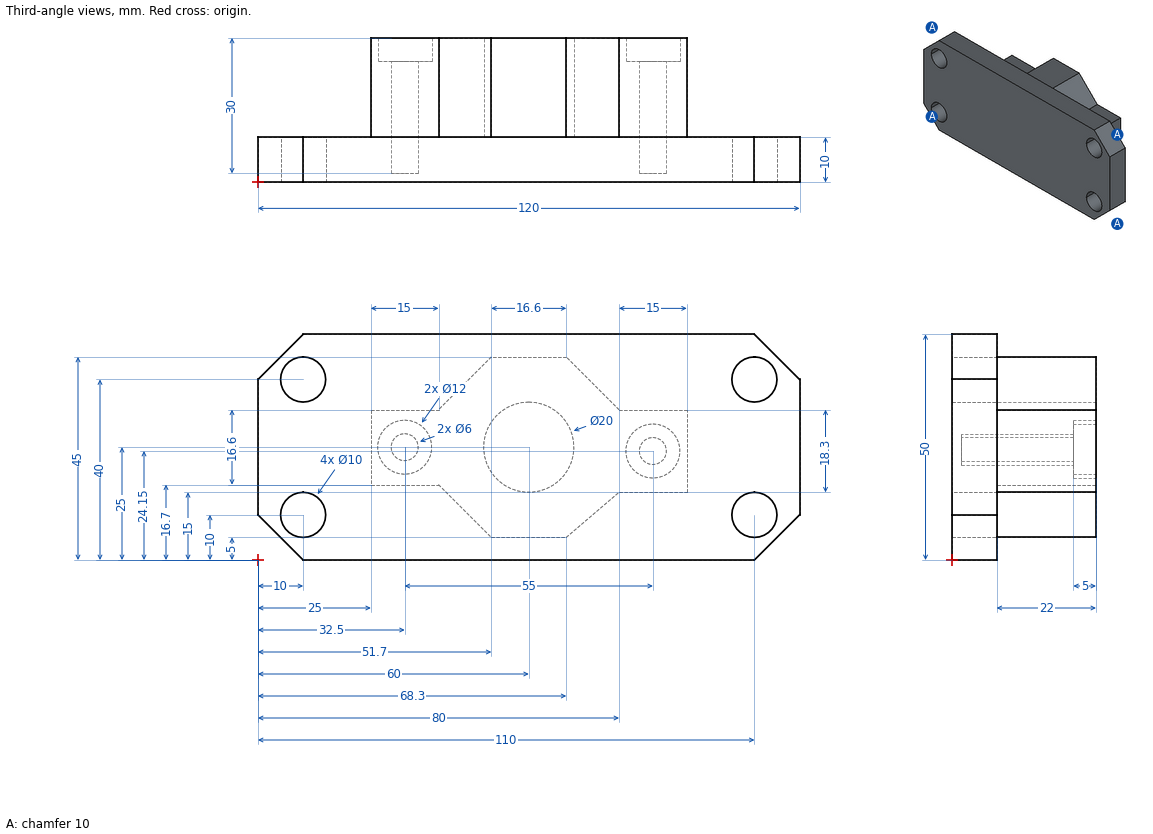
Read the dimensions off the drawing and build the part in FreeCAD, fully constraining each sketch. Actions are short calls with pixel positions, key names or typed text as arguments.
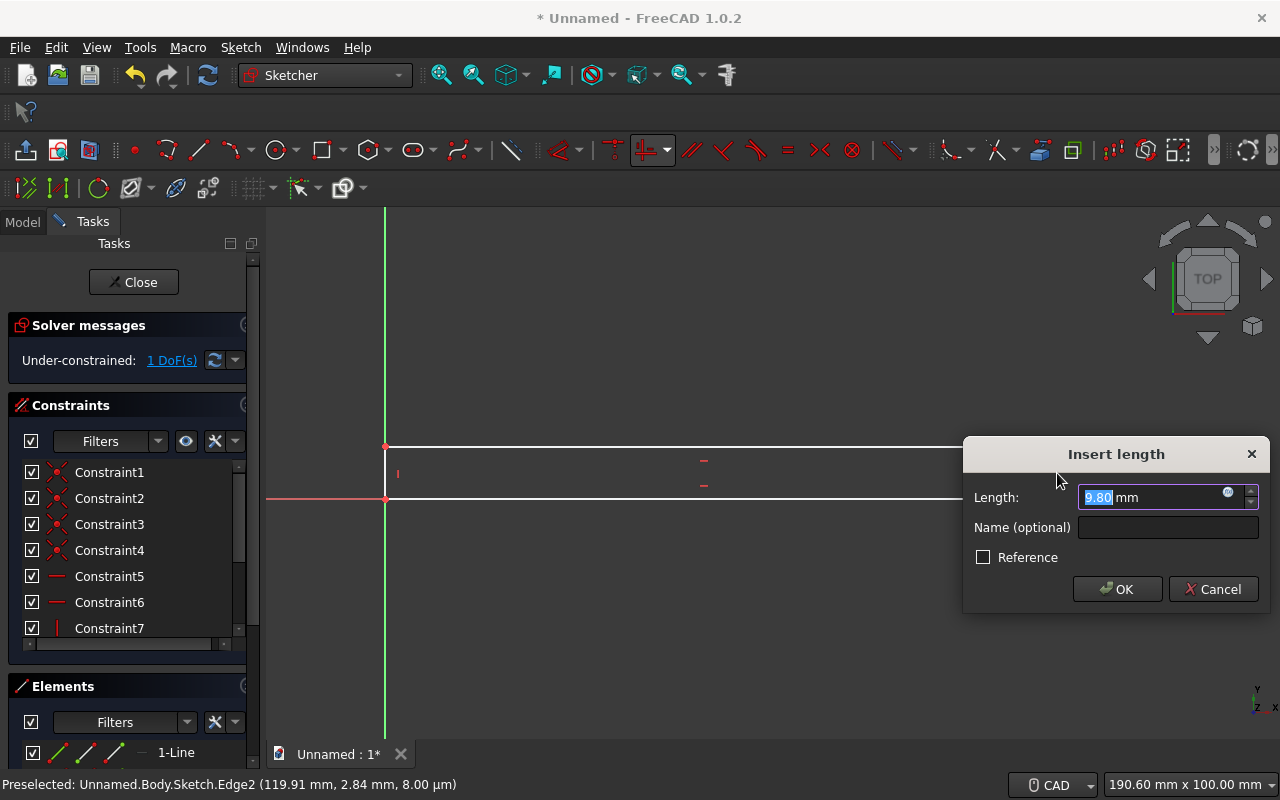
text(10)
key(Return)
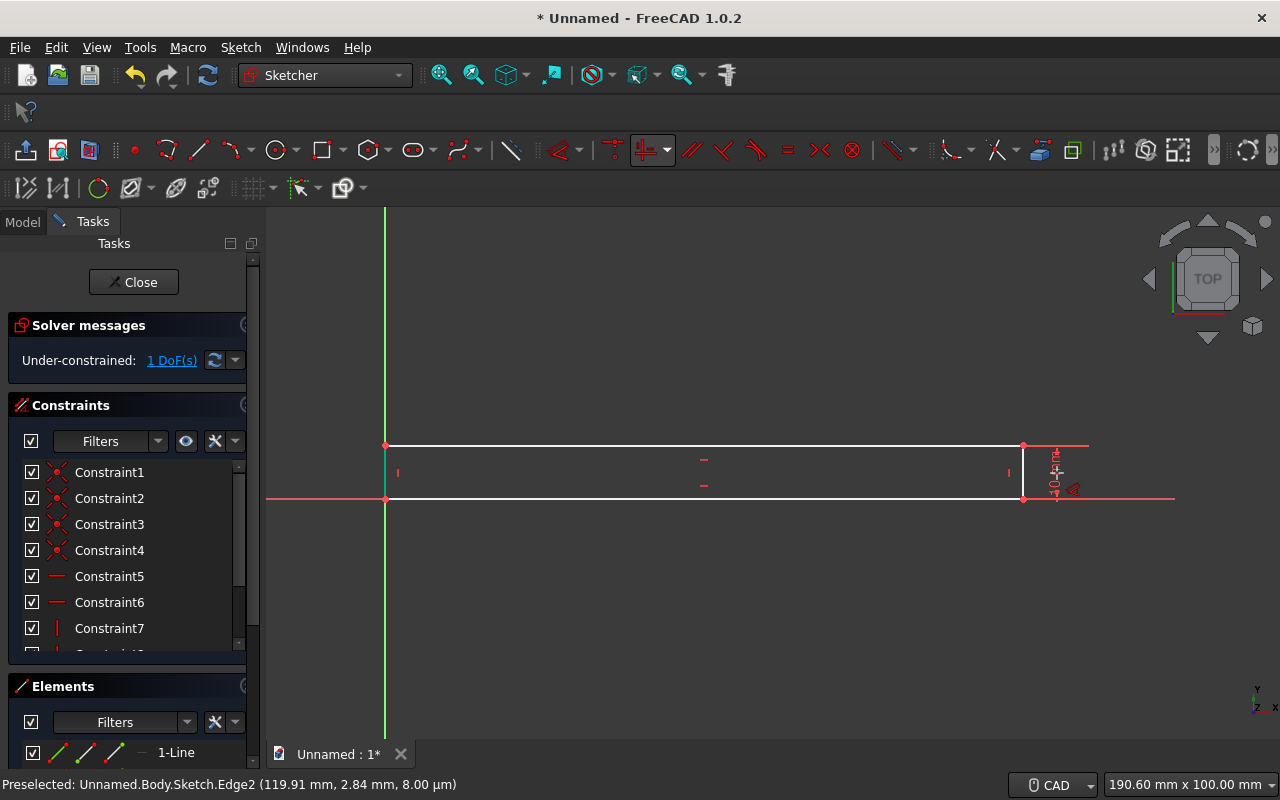
click(576, 499)
click(704, 533)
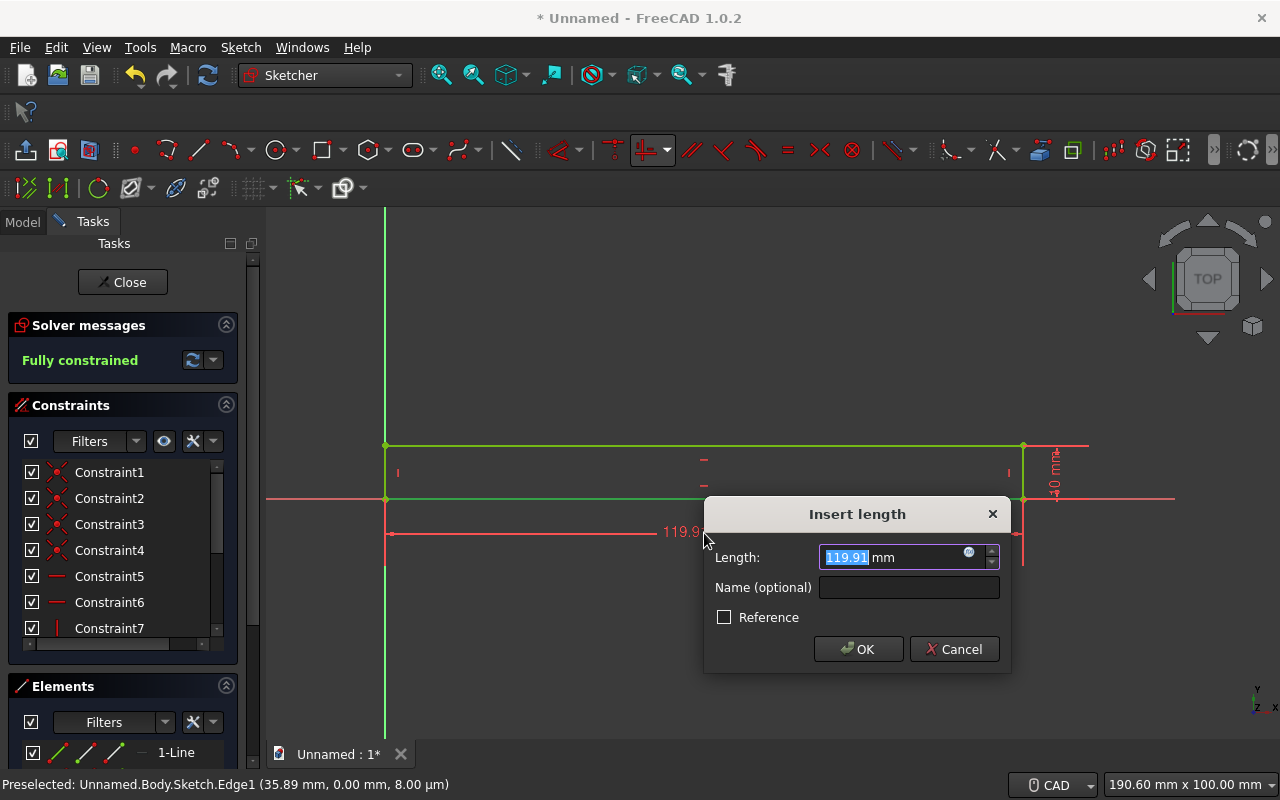
text(120)
key(Return)
key(Escape)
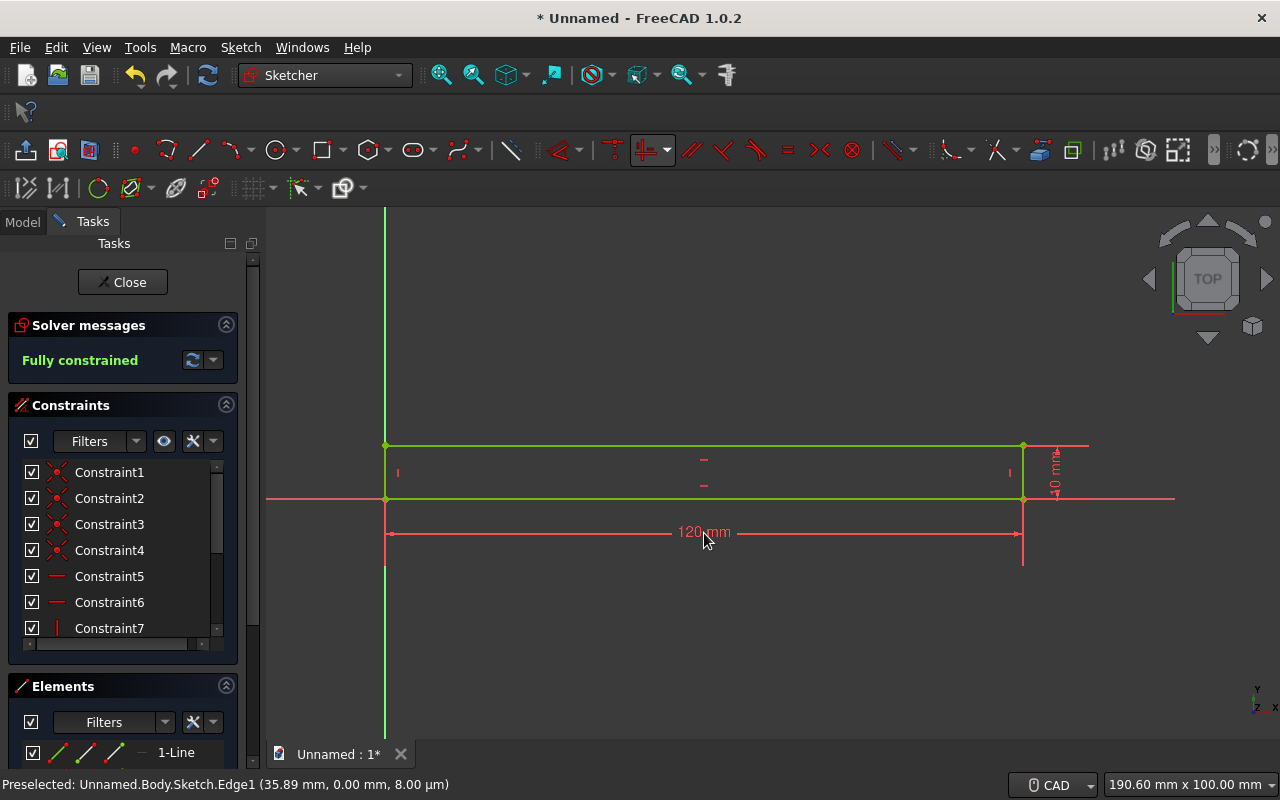
click(123, 282)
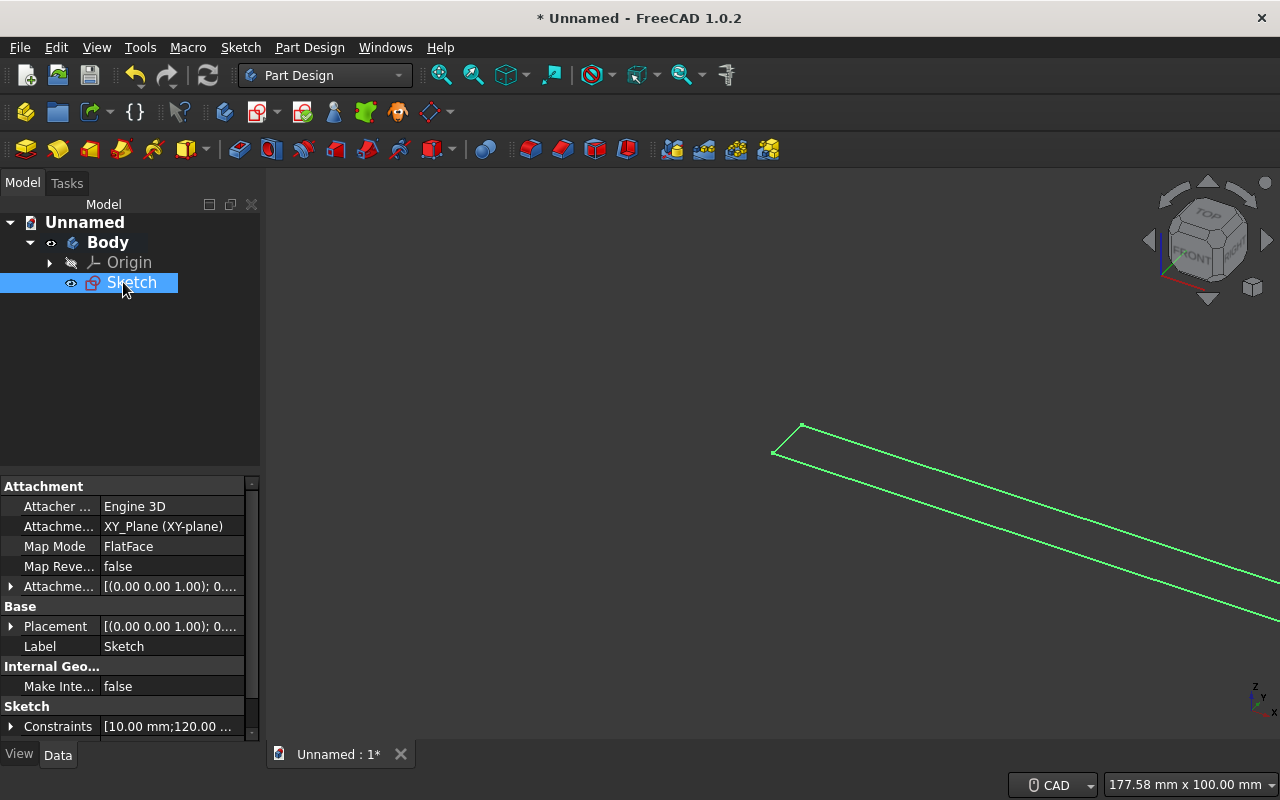
click(26, 150)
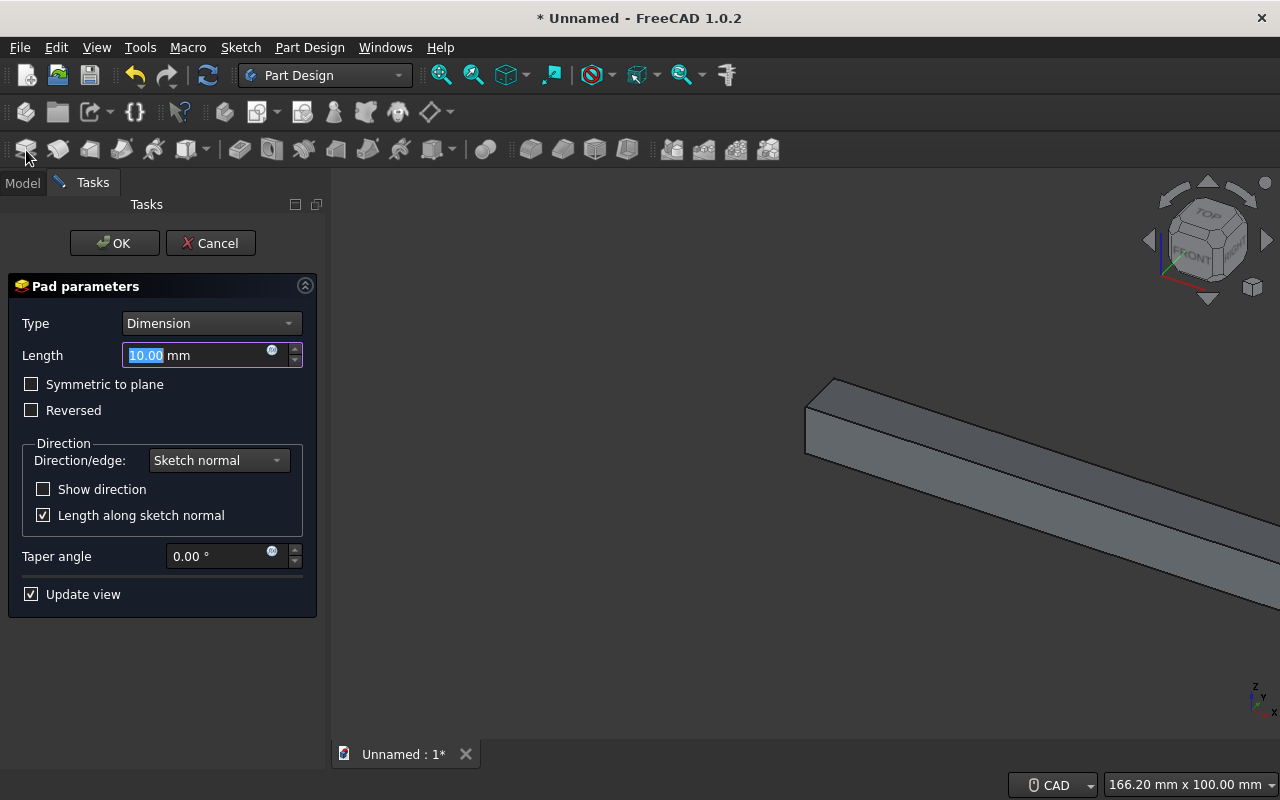
text(50)
key(Tab)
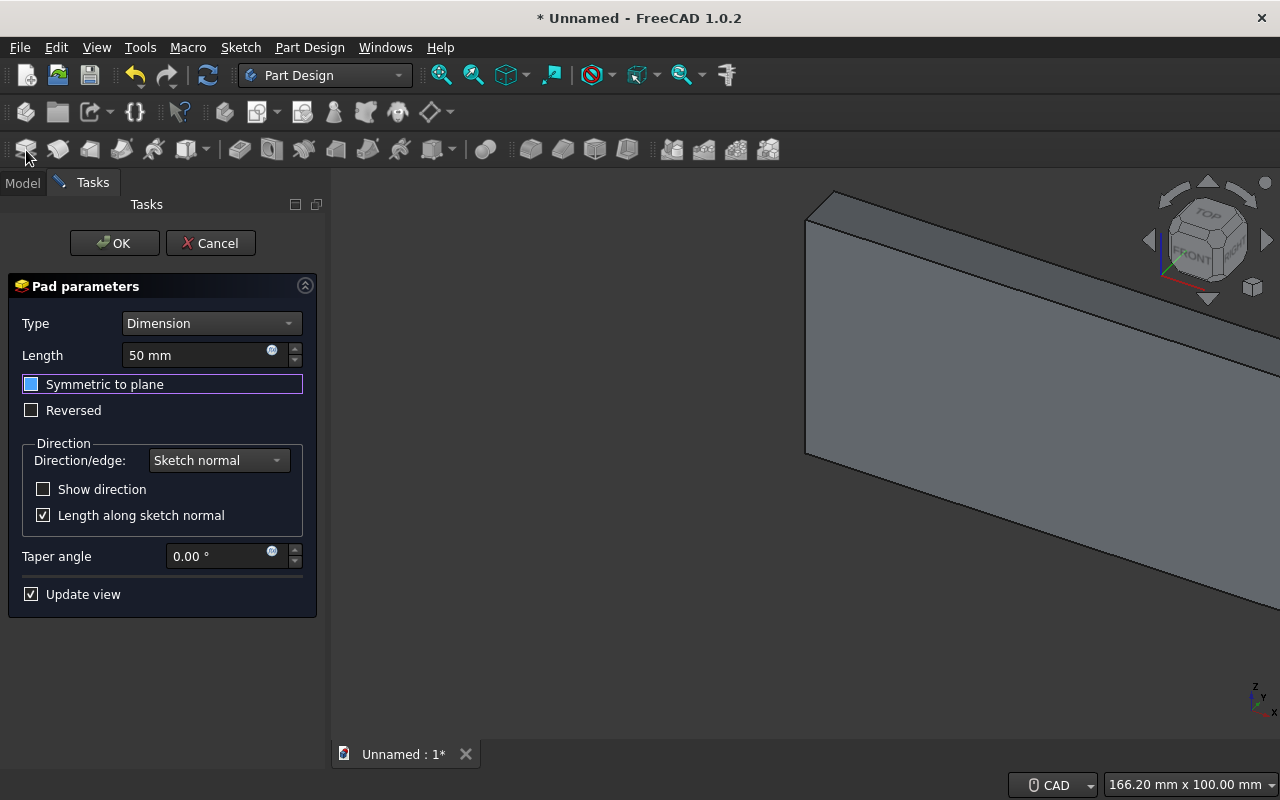
click(115, 243)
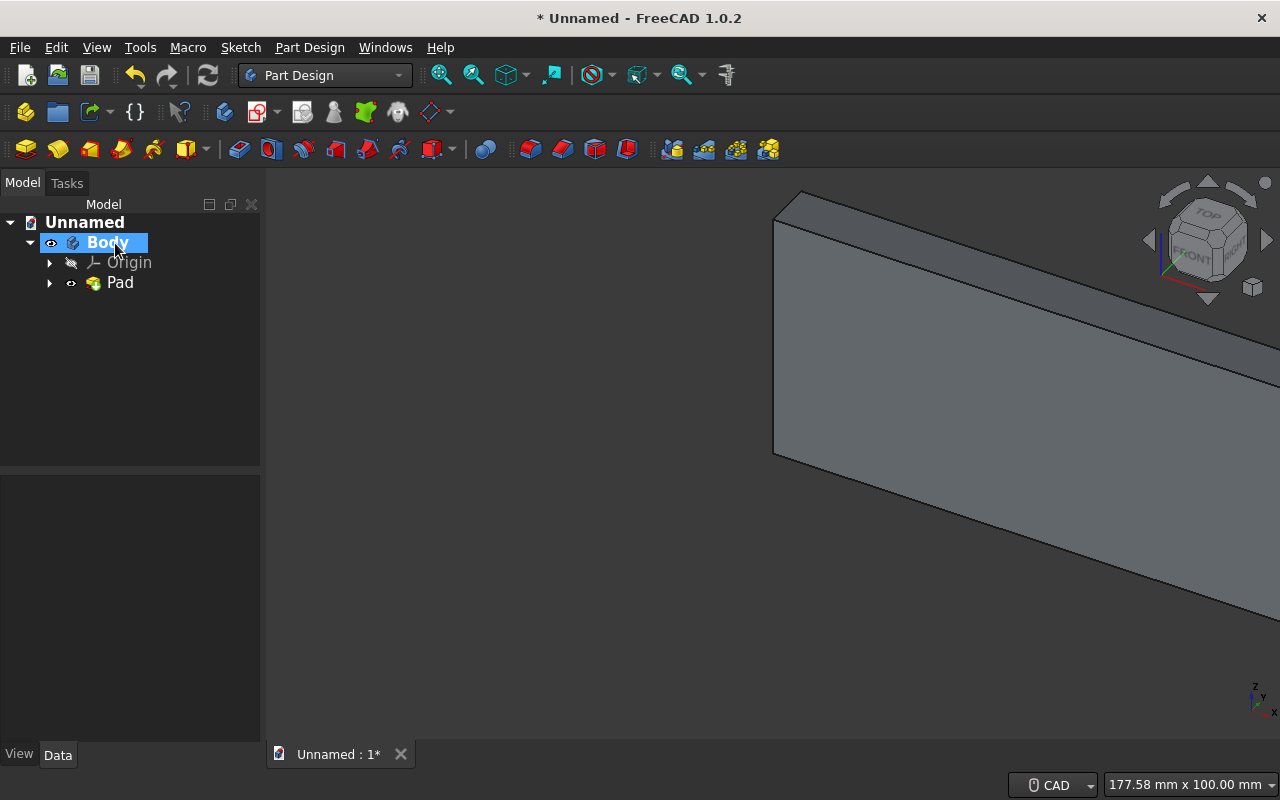
click(442, 76)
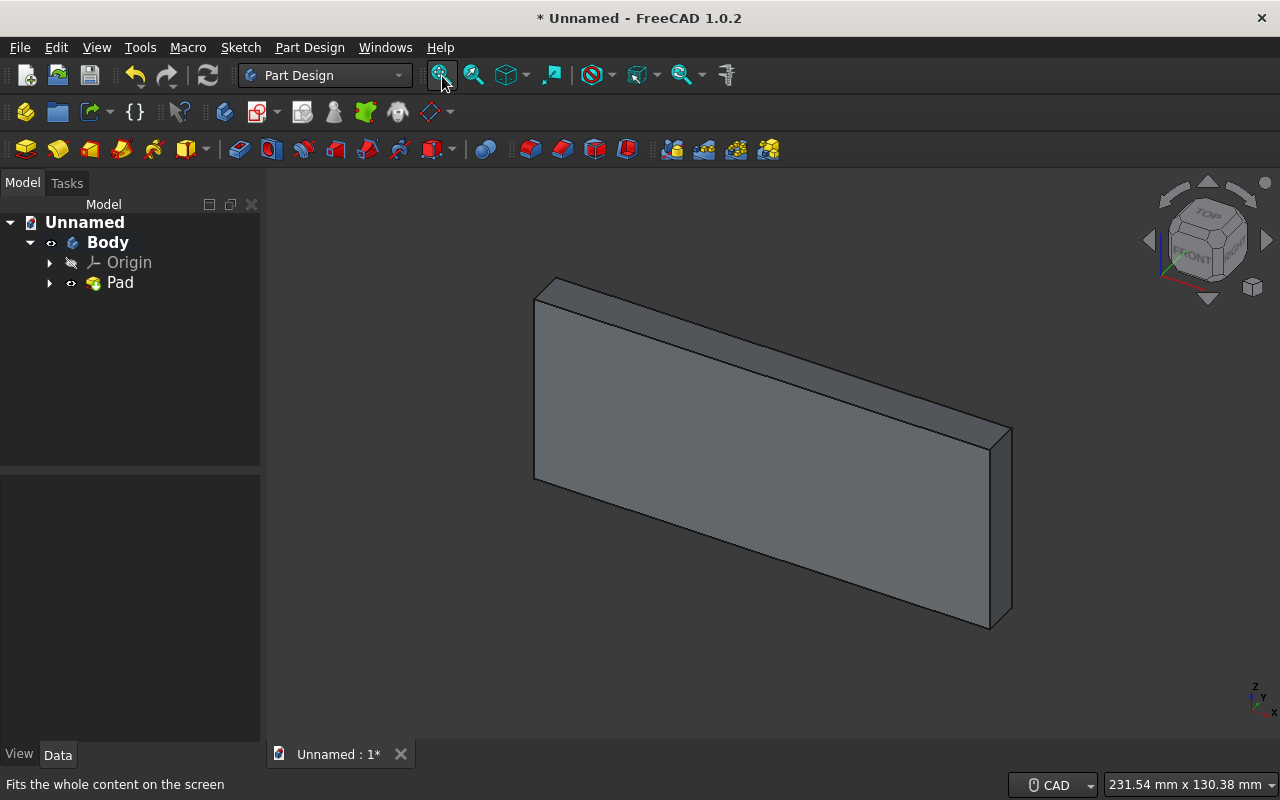
key(4)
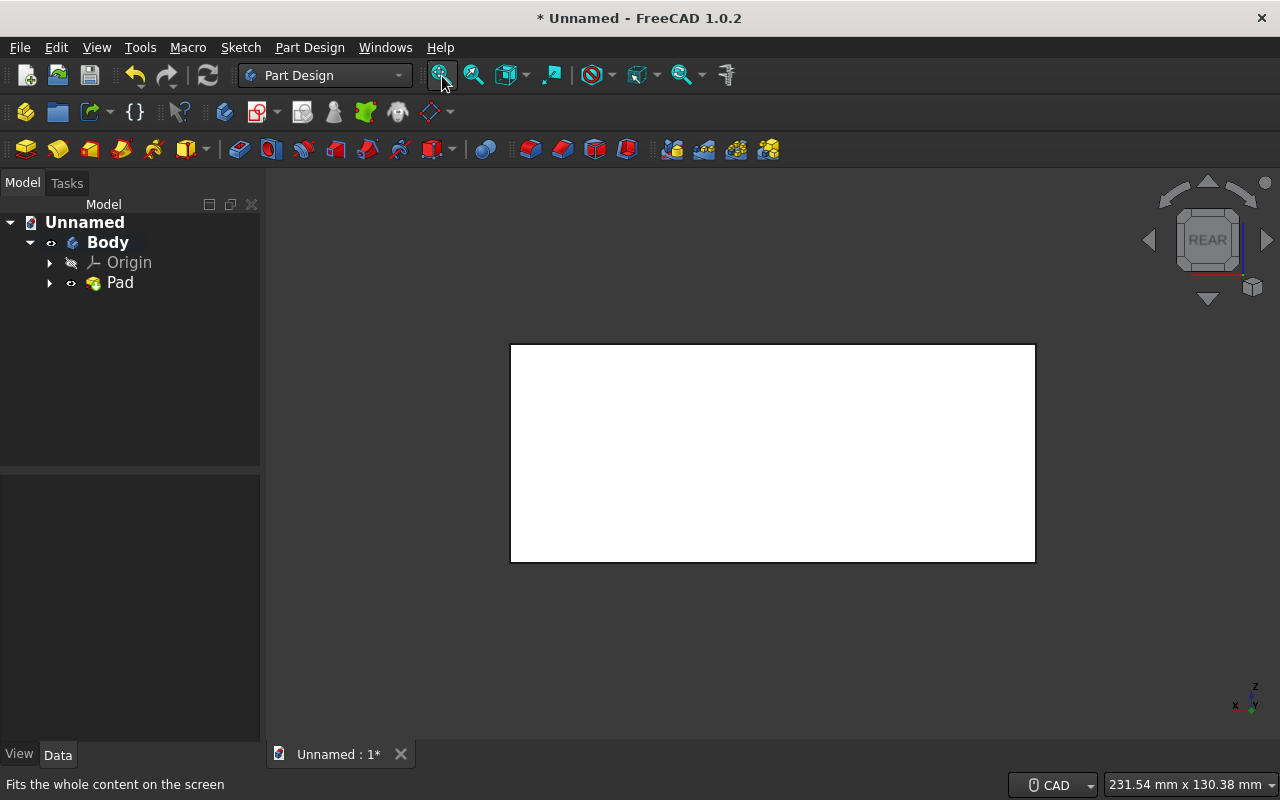
click(623, 452)